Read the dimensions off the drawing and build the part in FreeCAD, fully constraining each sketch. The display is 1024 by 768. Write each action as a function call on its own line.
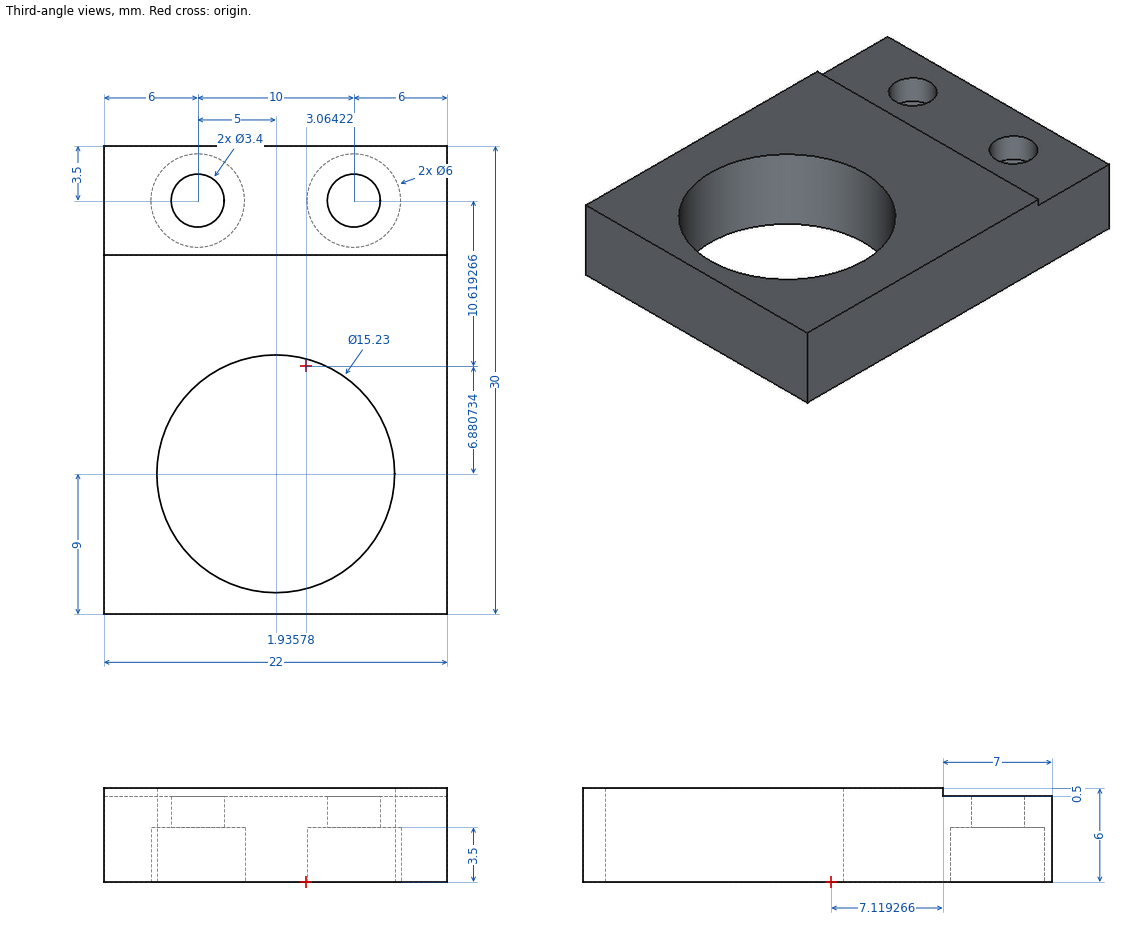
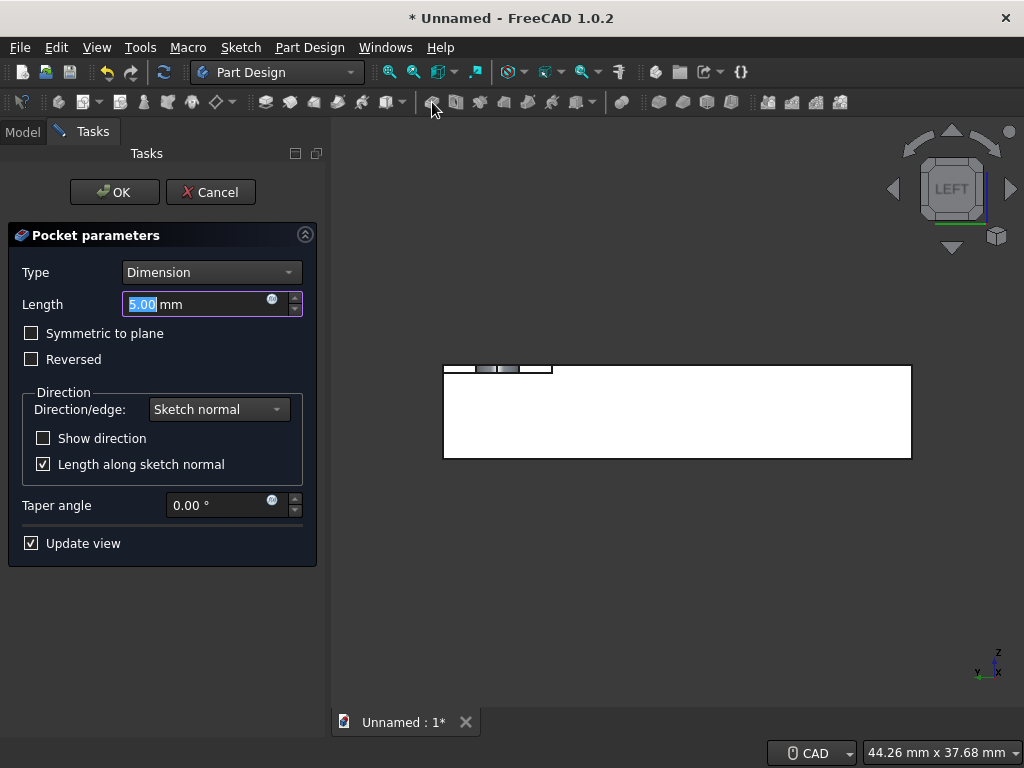
click(212, 272)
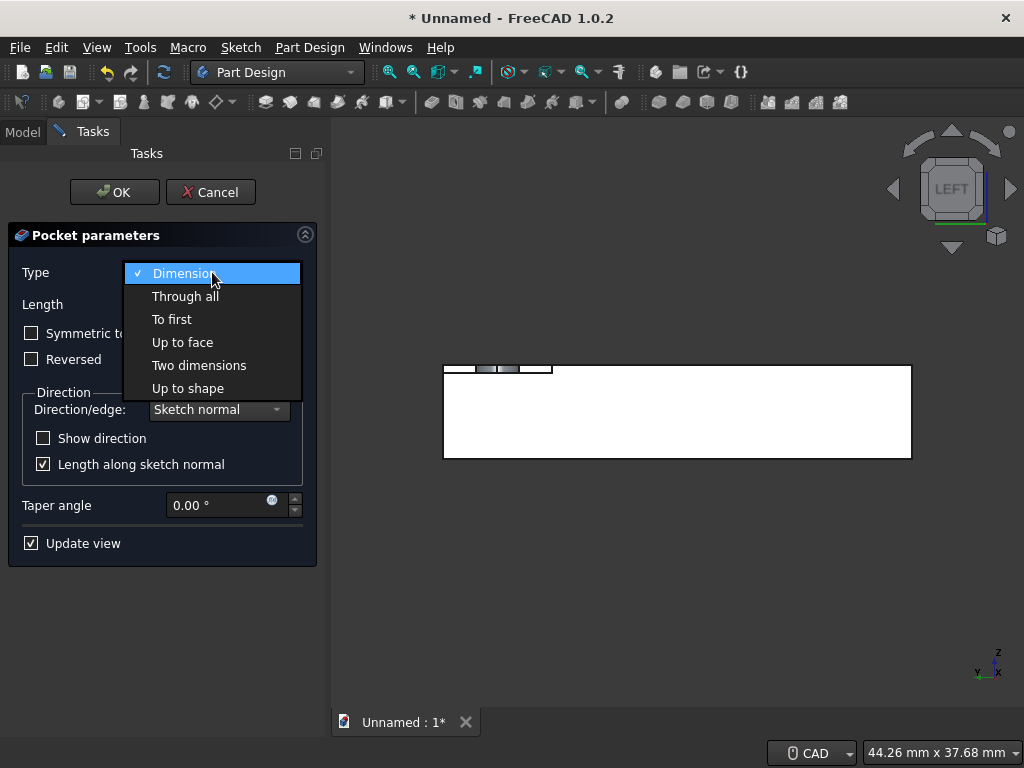
click(212, 296)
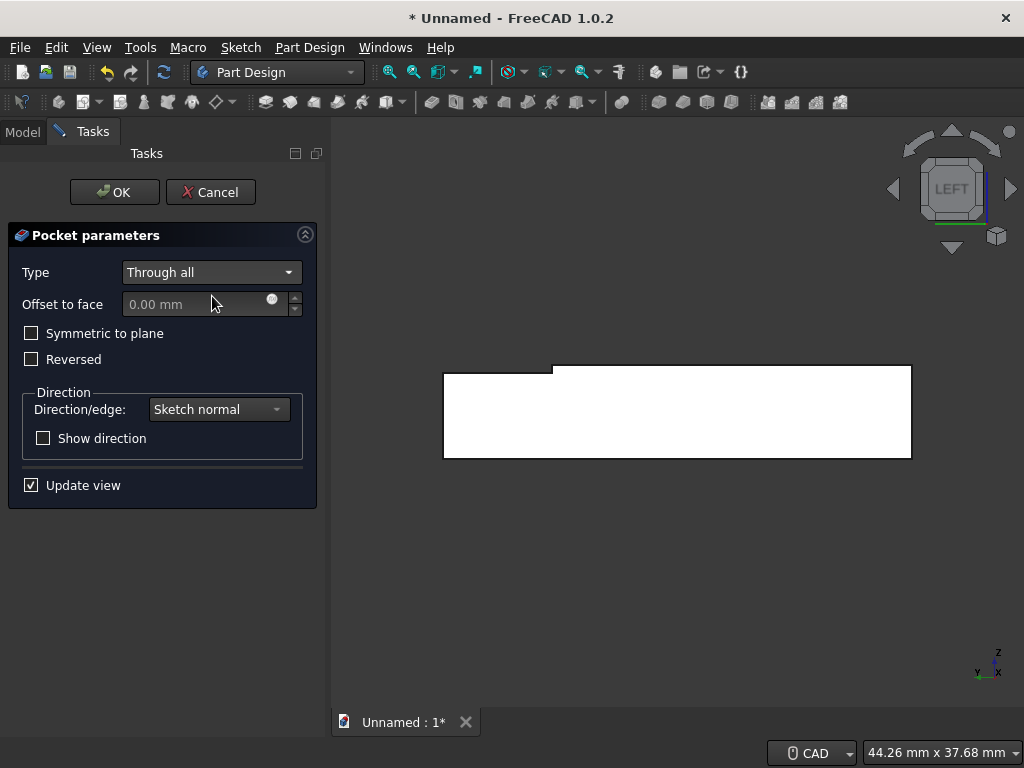
click(115, 192)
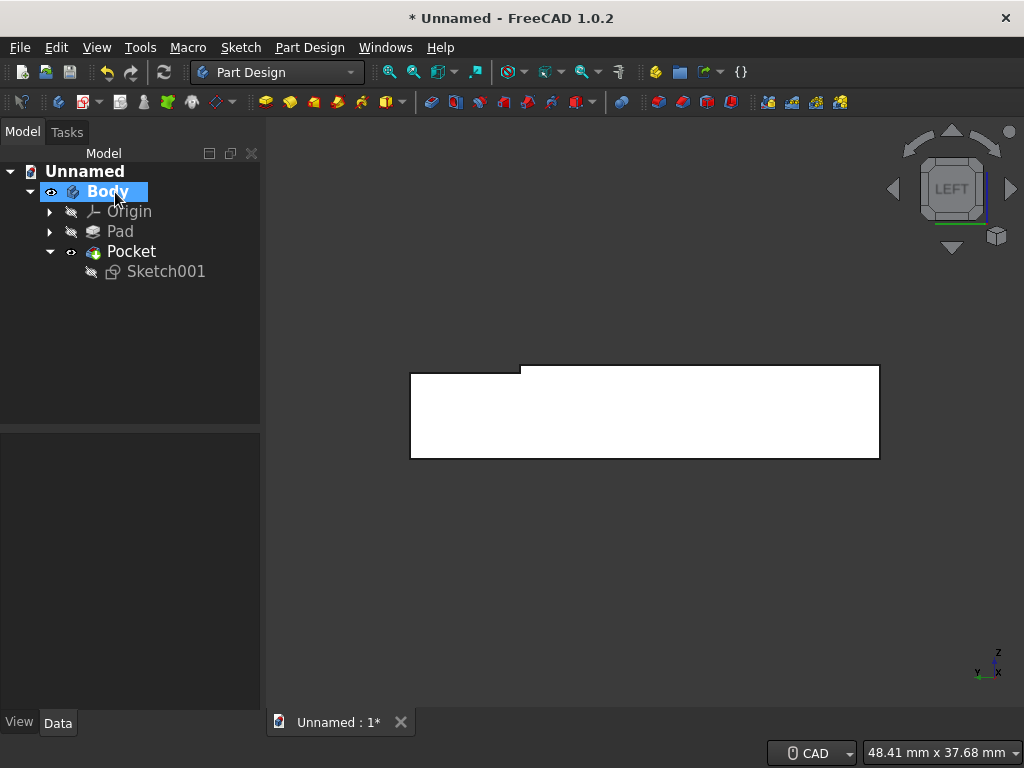
click(84, 102)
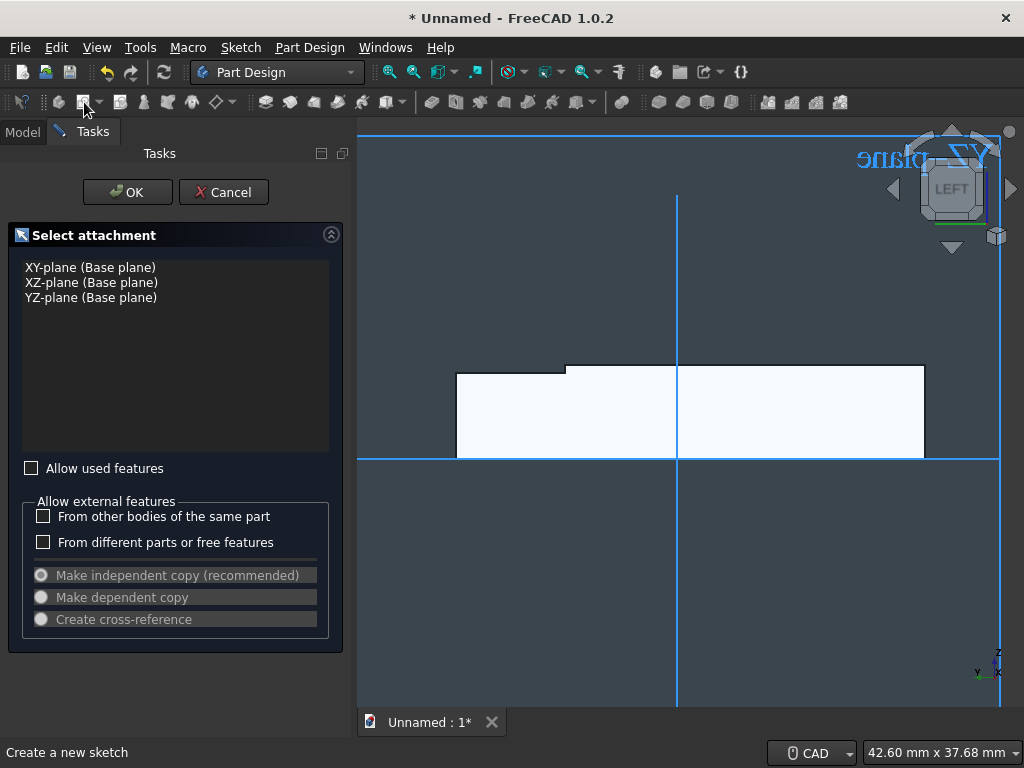
click(82, 268)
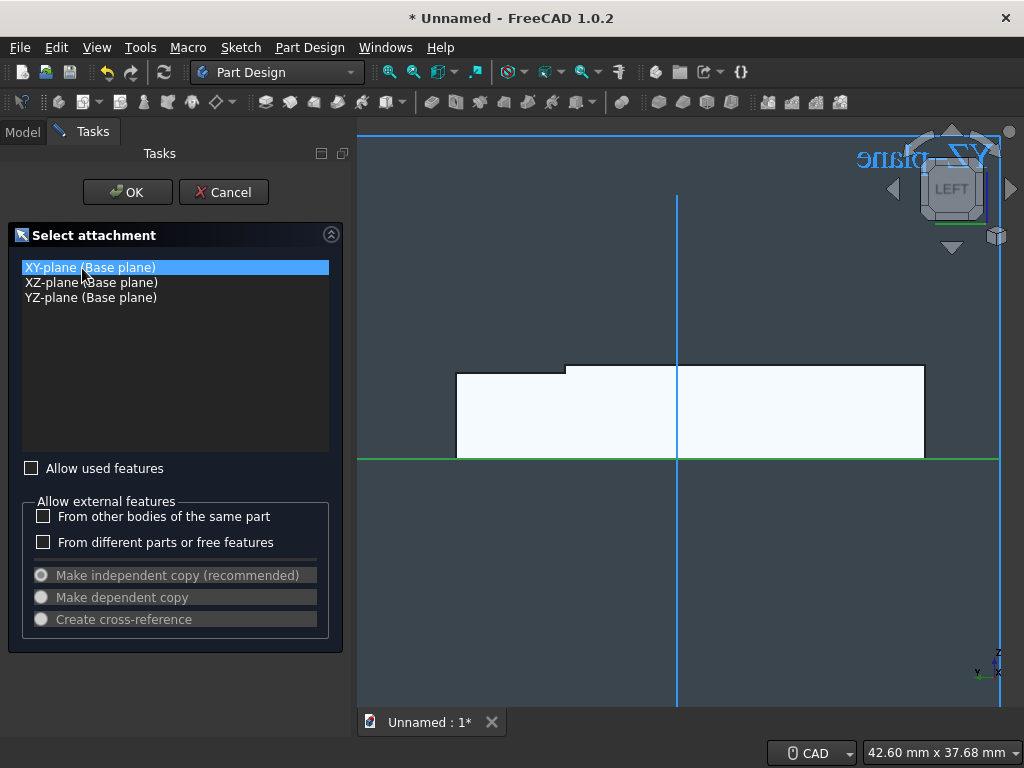
click(128, 192)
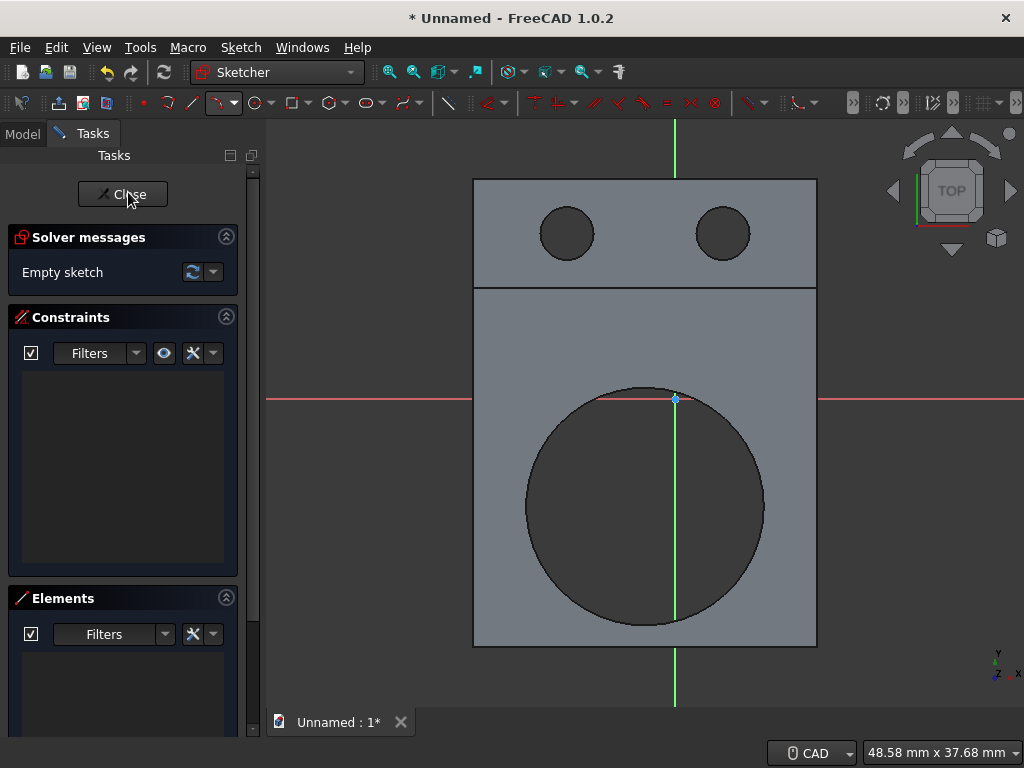
key(q)
key(s)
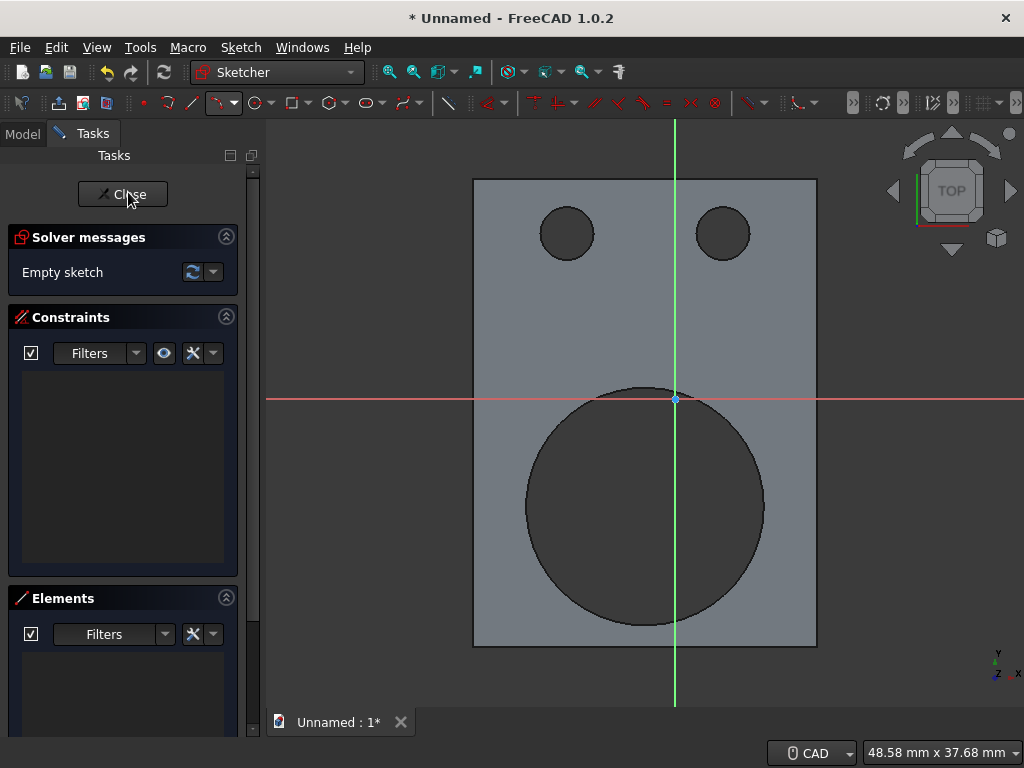
scroll(784, 147, up, 2)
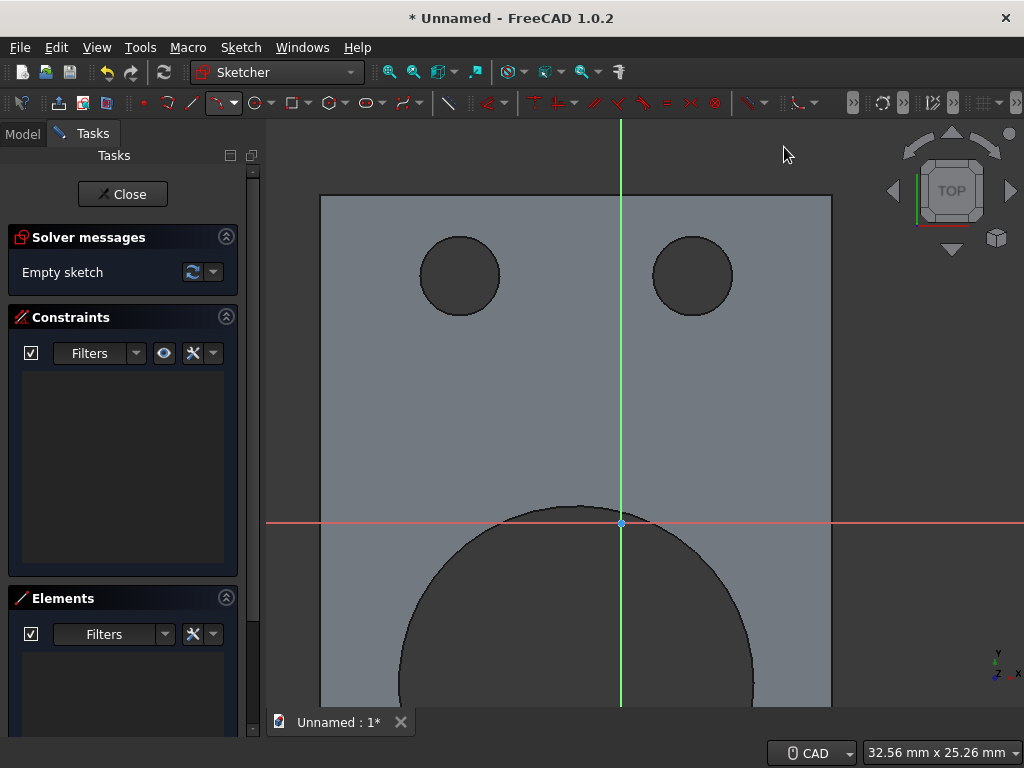
key(g)
key(c)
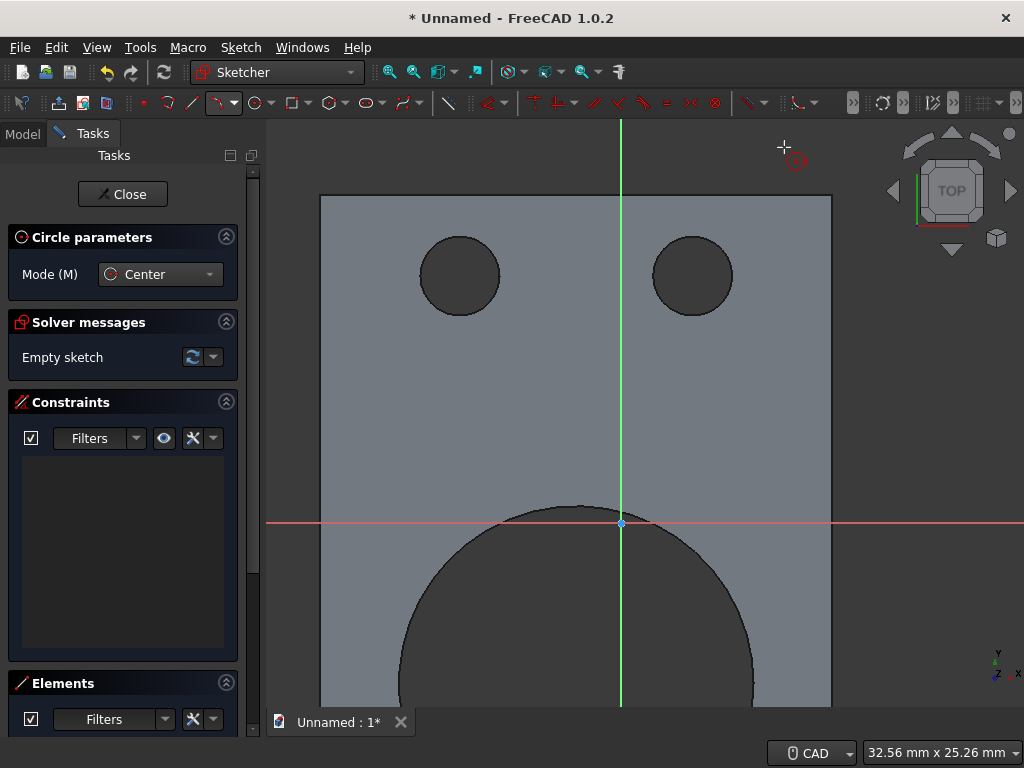
click(693, 276)
move(742, 227)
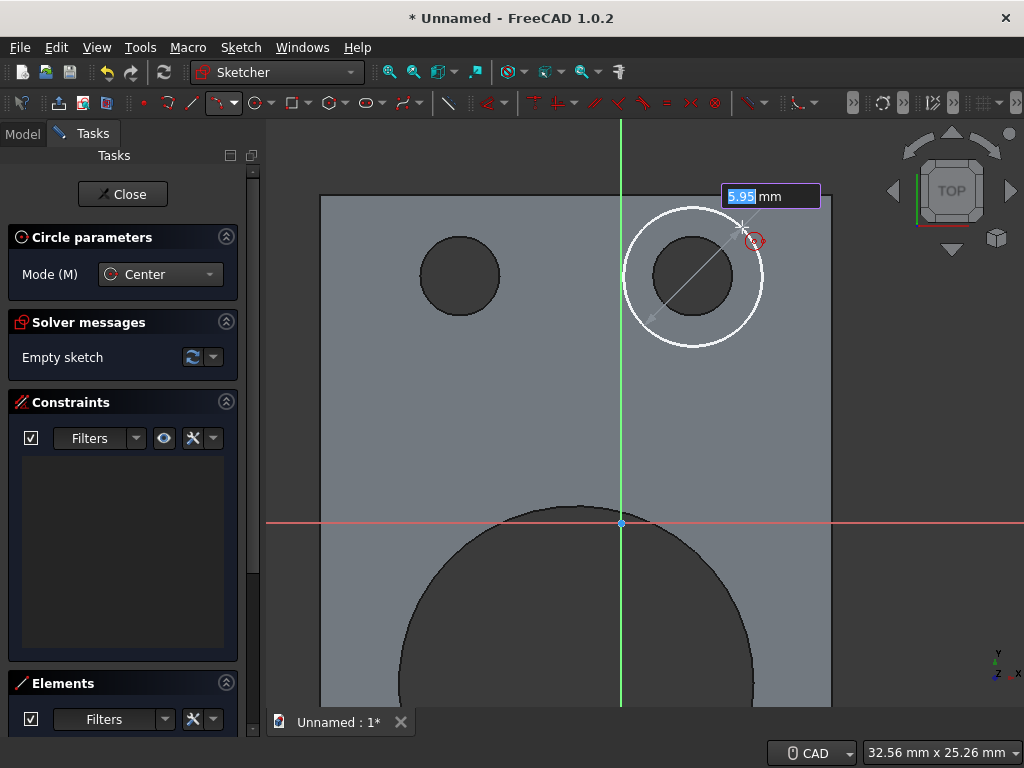
text(6)
key(Return)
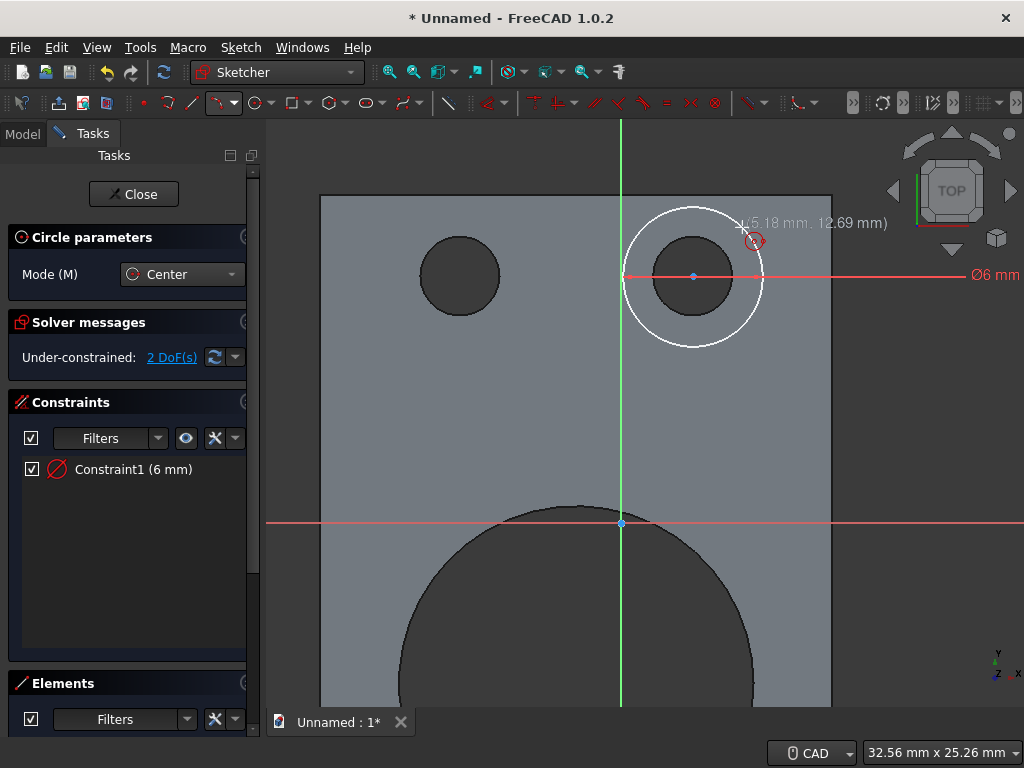
click(460, 276)
move(509, 227)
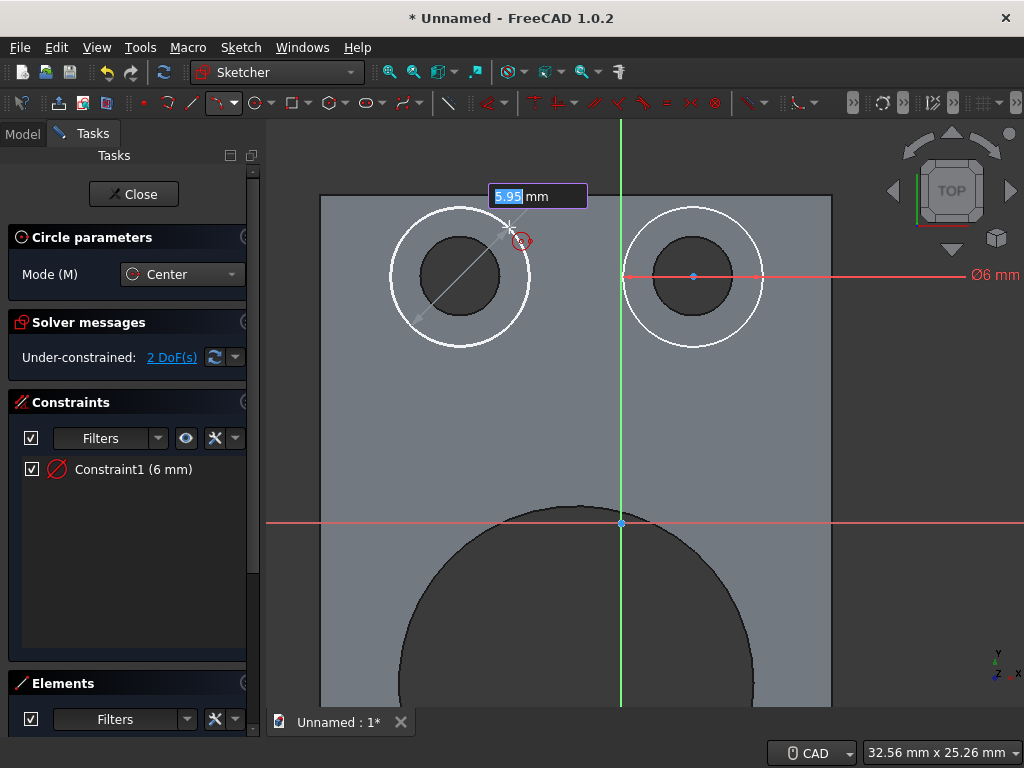
text(6)
key(Return)
key(Escape)